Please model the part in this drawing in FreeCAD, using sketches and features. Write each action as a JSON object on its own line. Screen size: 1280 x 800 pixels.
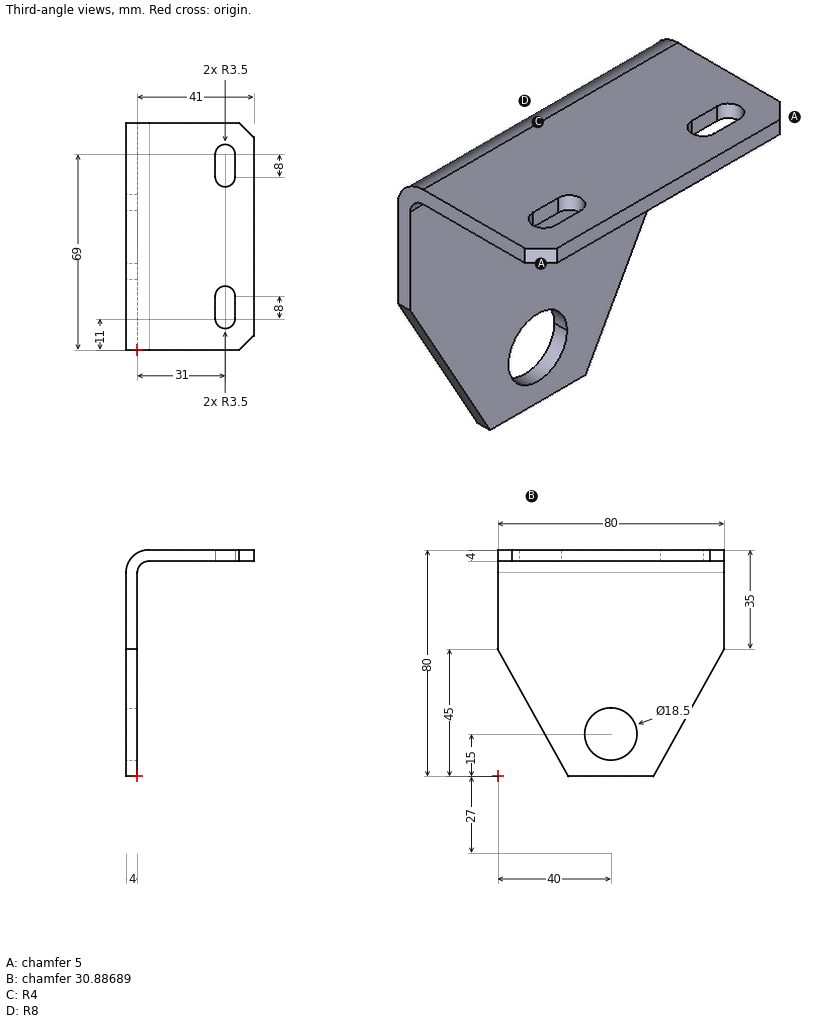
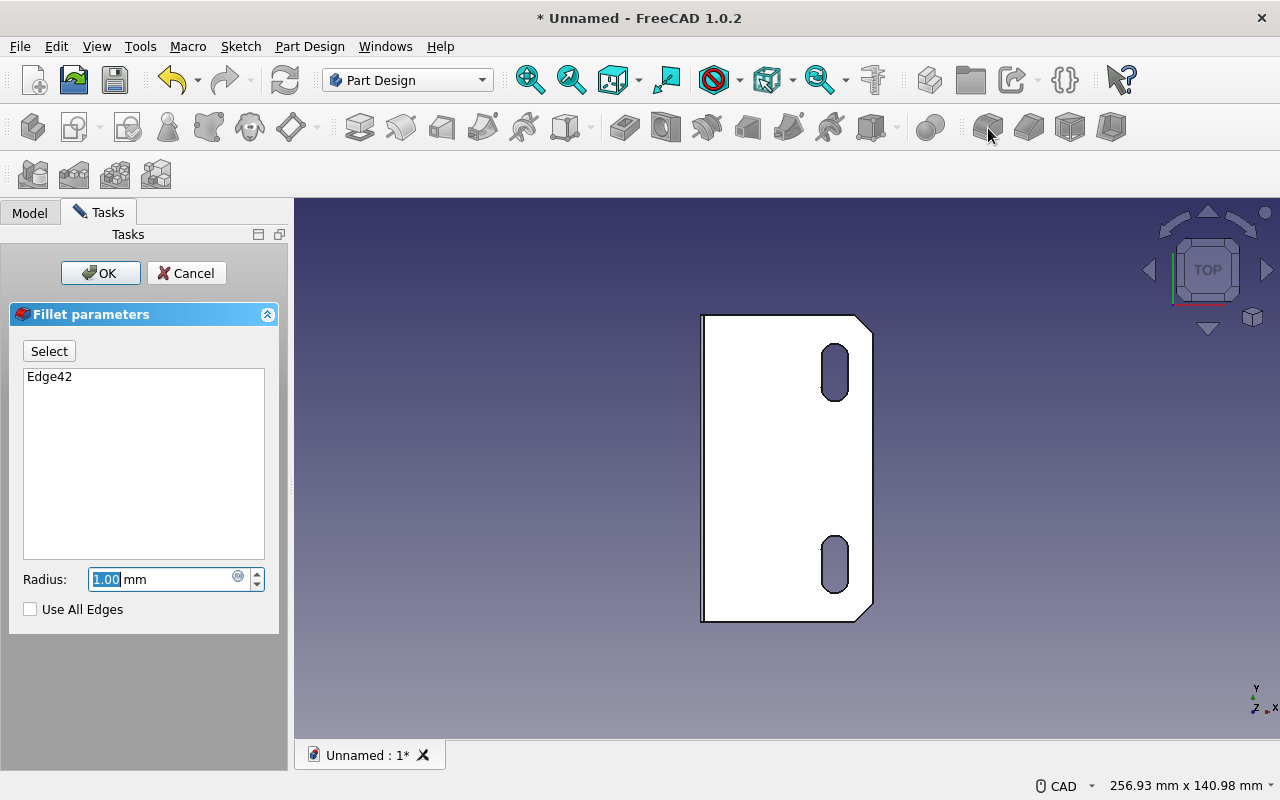
{"action": "type", "text": "8"}
{"action": "key", "text": "Tab"}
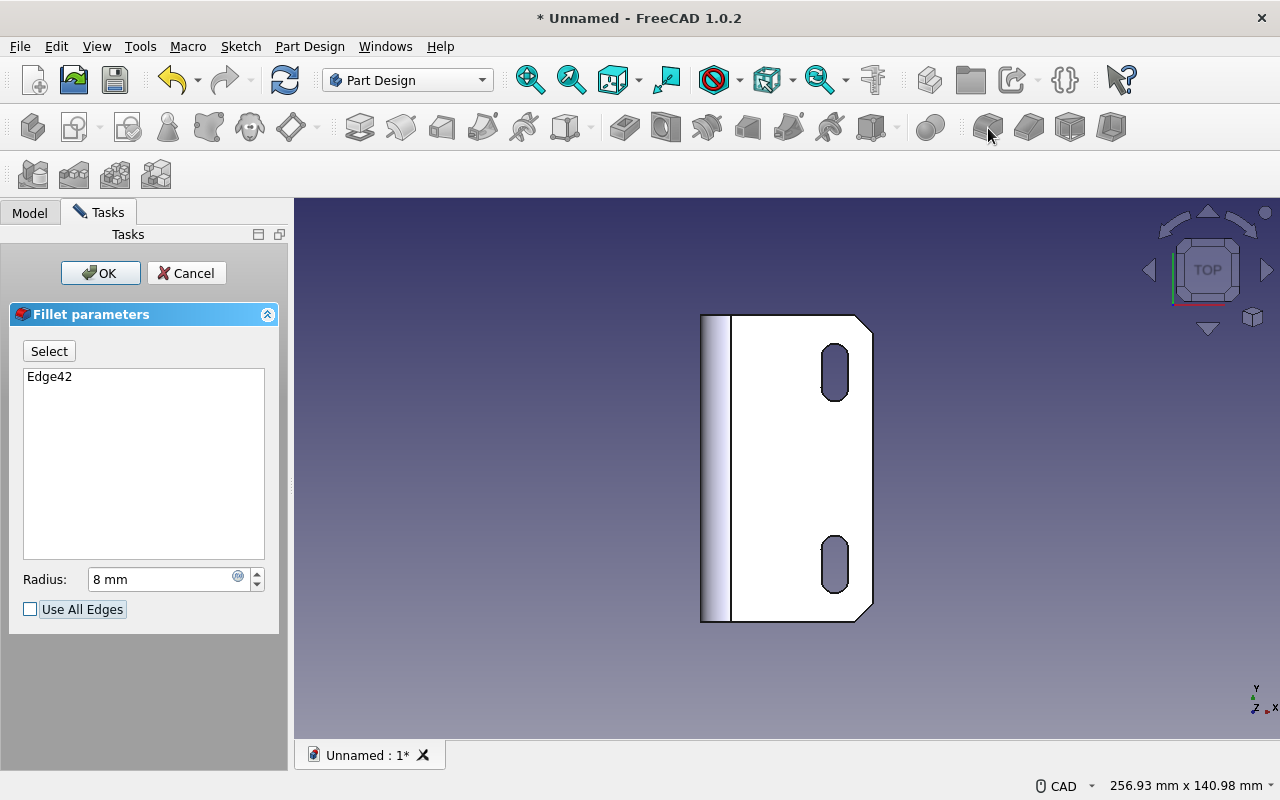
{"action": "left_click", "coordinate": [101, 273]}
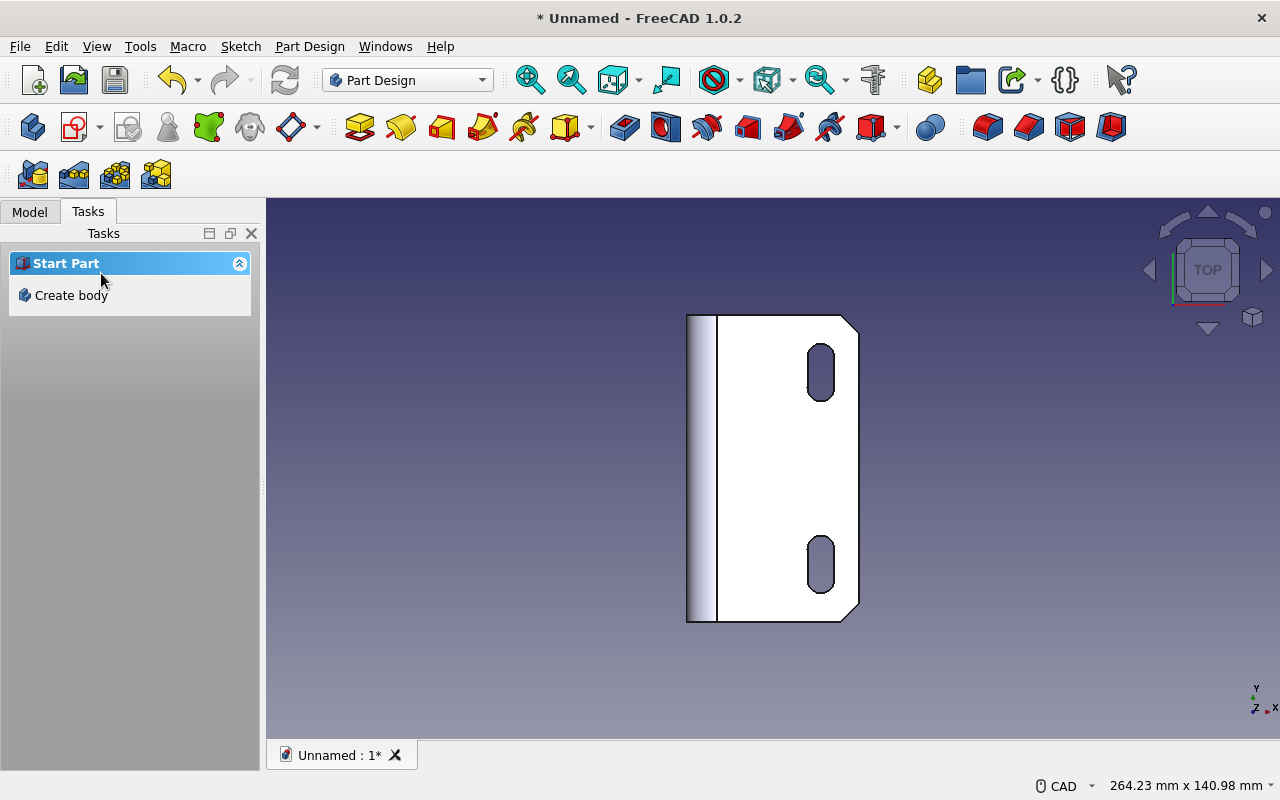
{"action": "key", "text": "0"}